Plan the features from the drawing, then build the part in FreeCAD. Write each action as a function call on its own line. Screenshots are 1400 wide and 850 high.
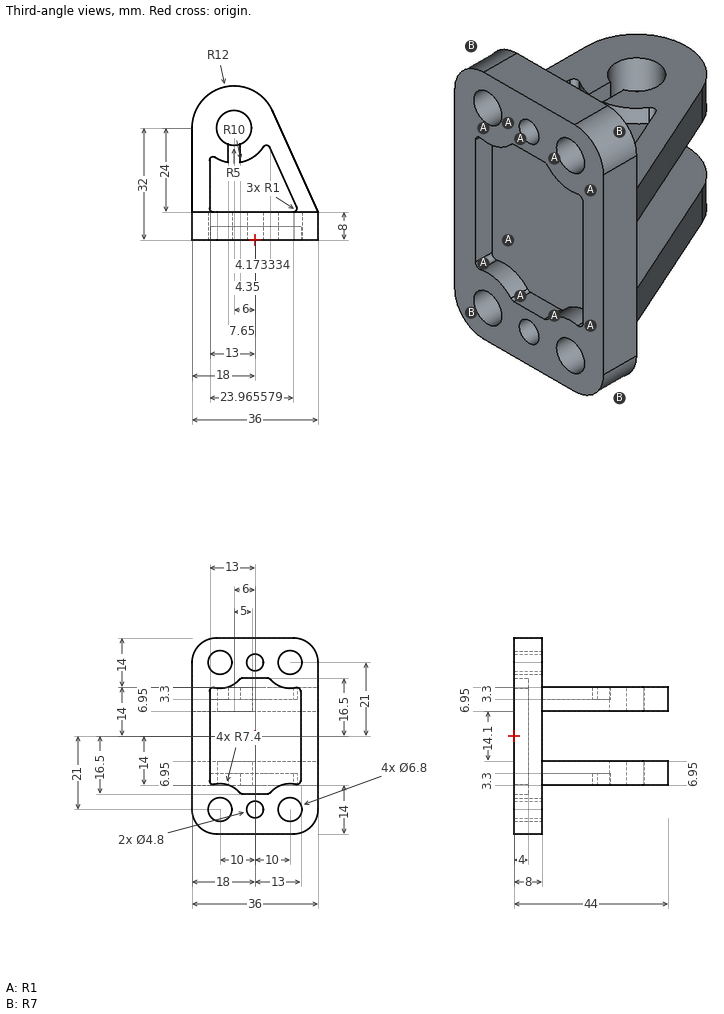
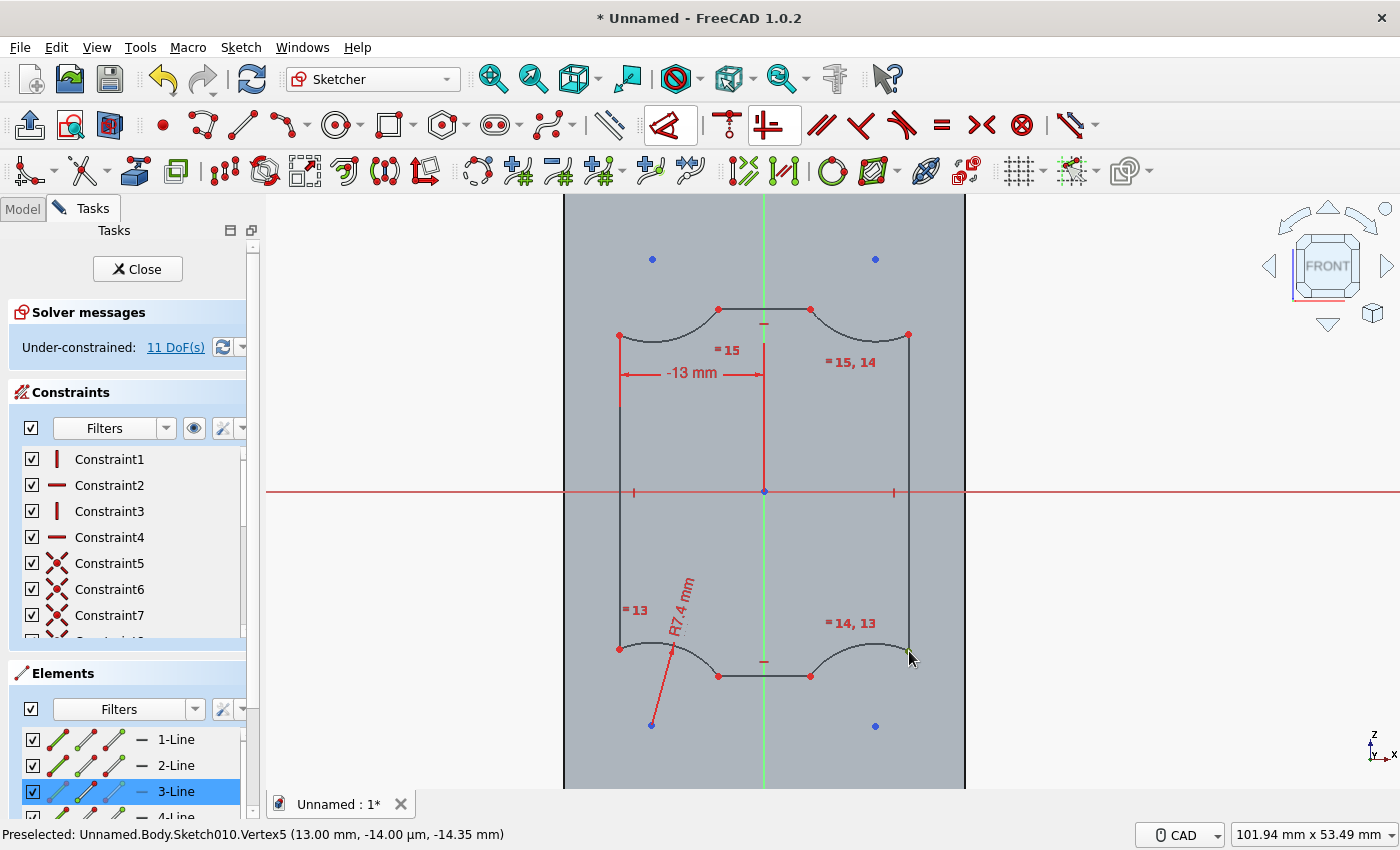
key(l)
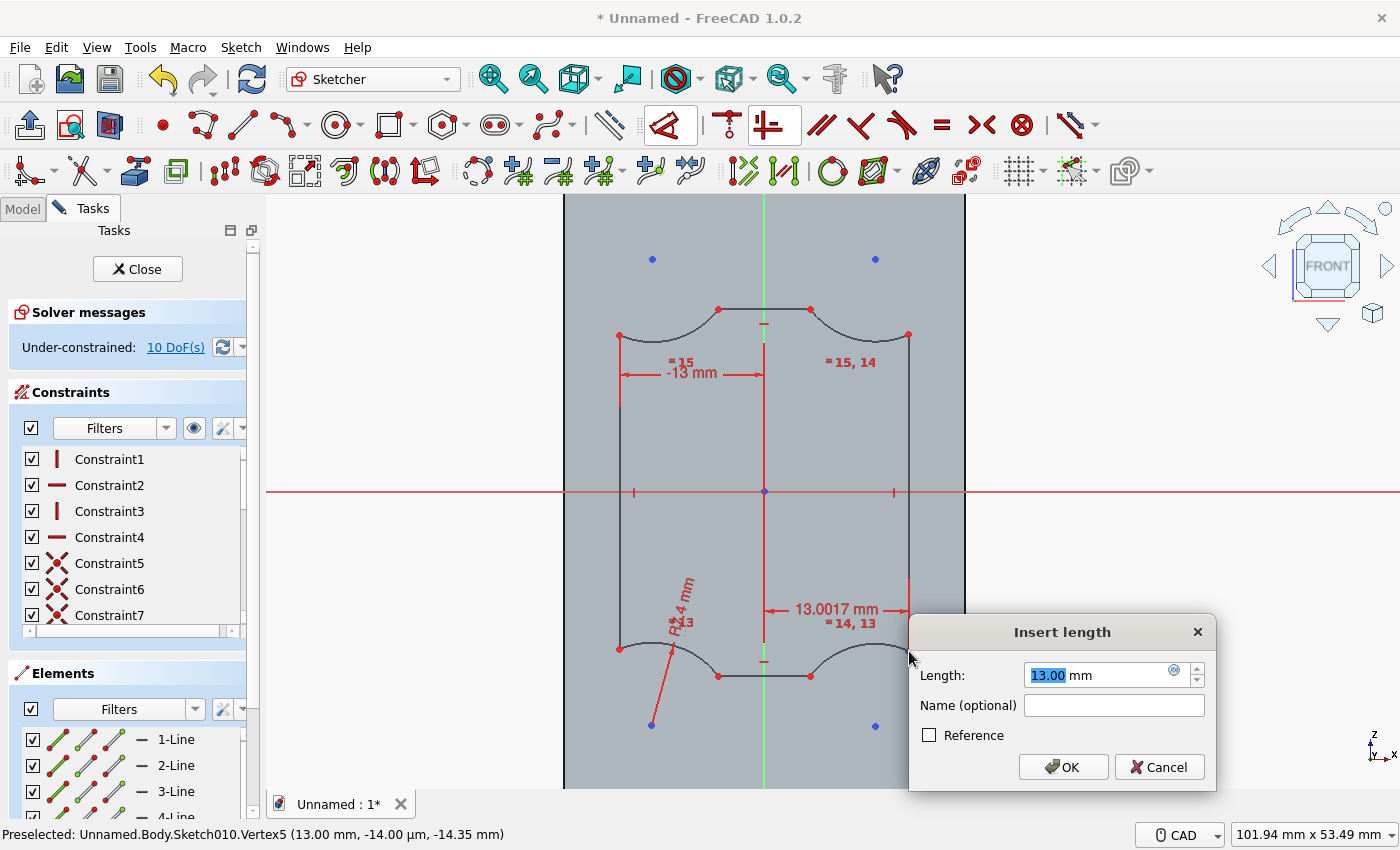
text(13)
key(Return)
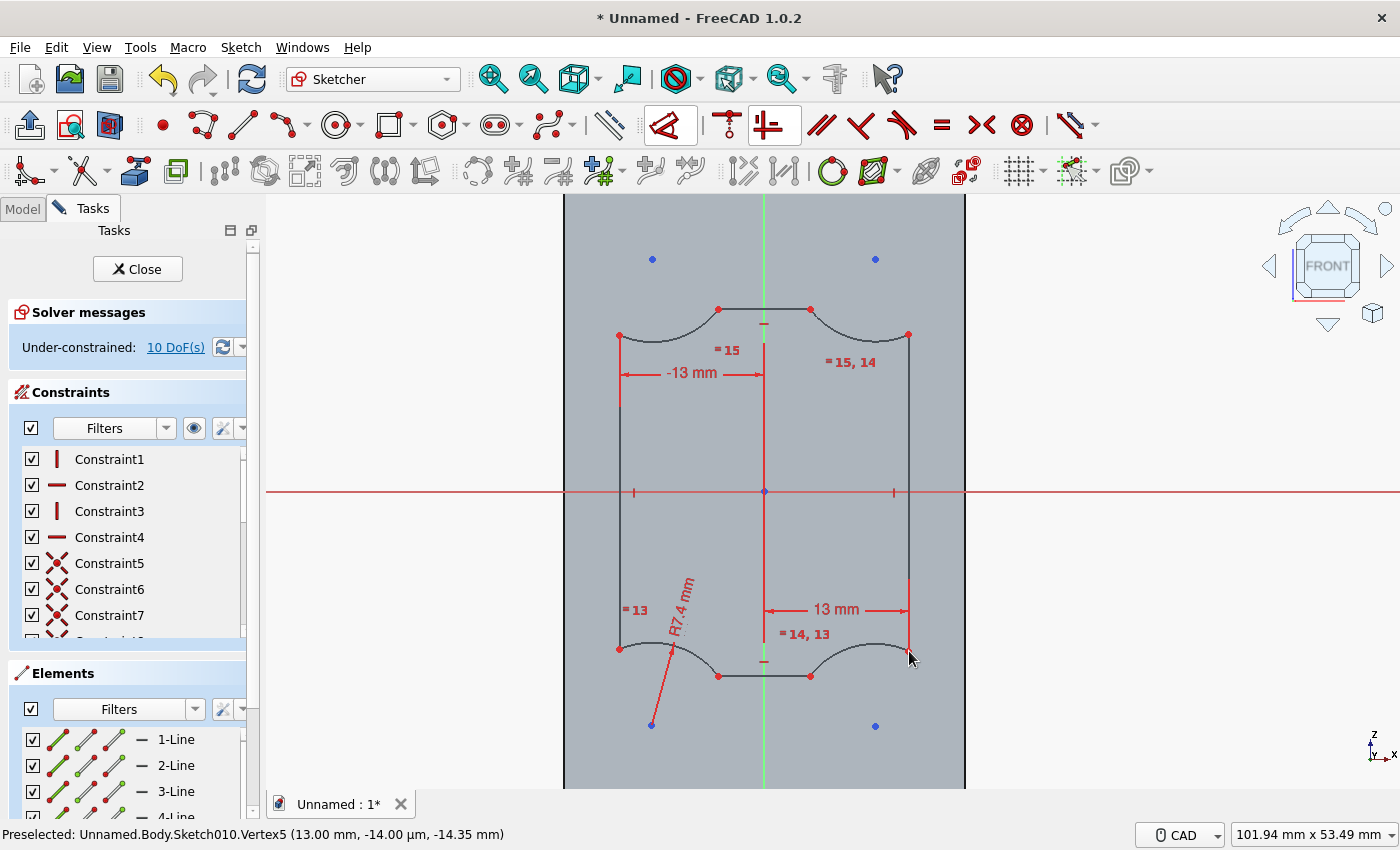
click(652, 725)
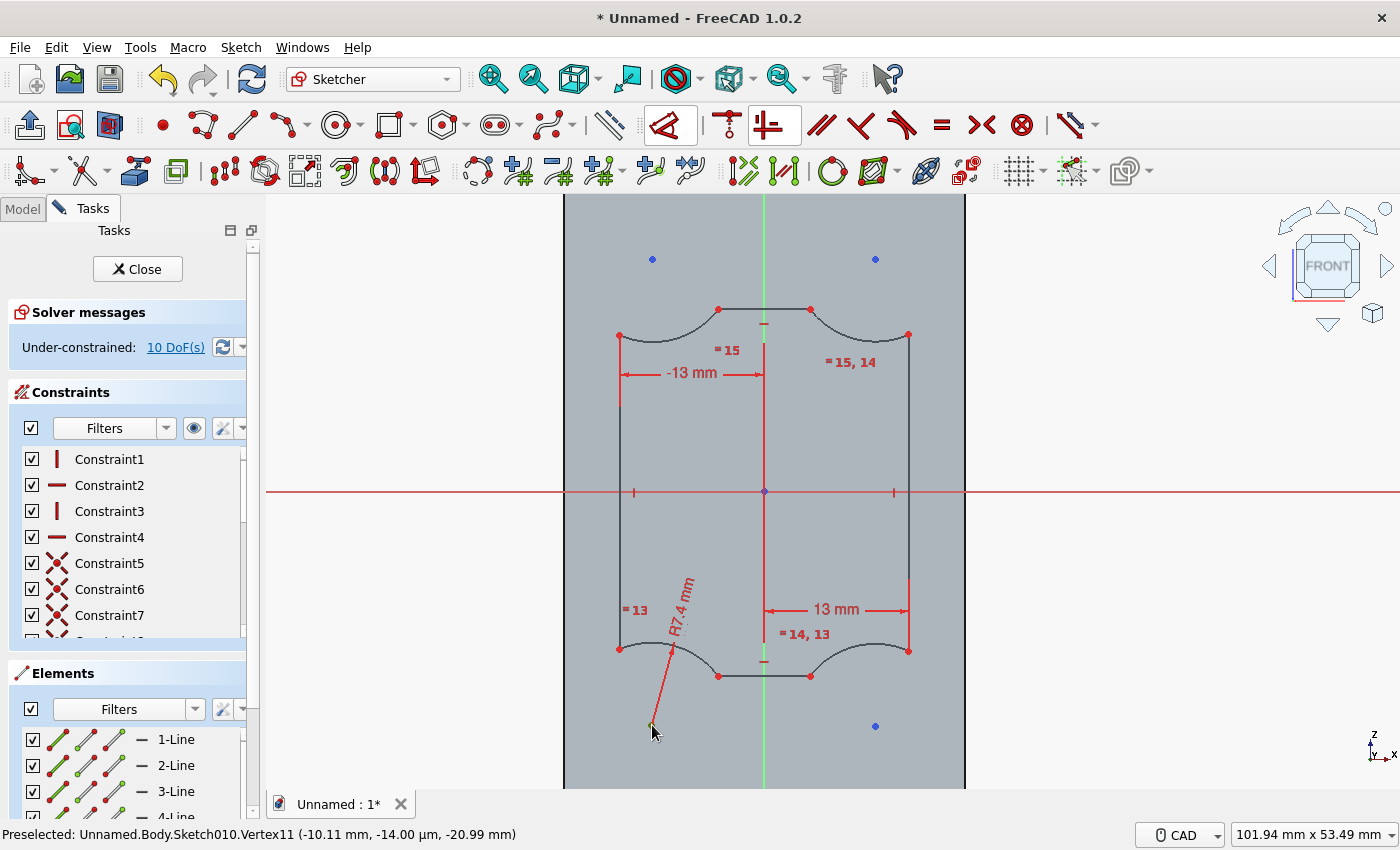
click(692, 126)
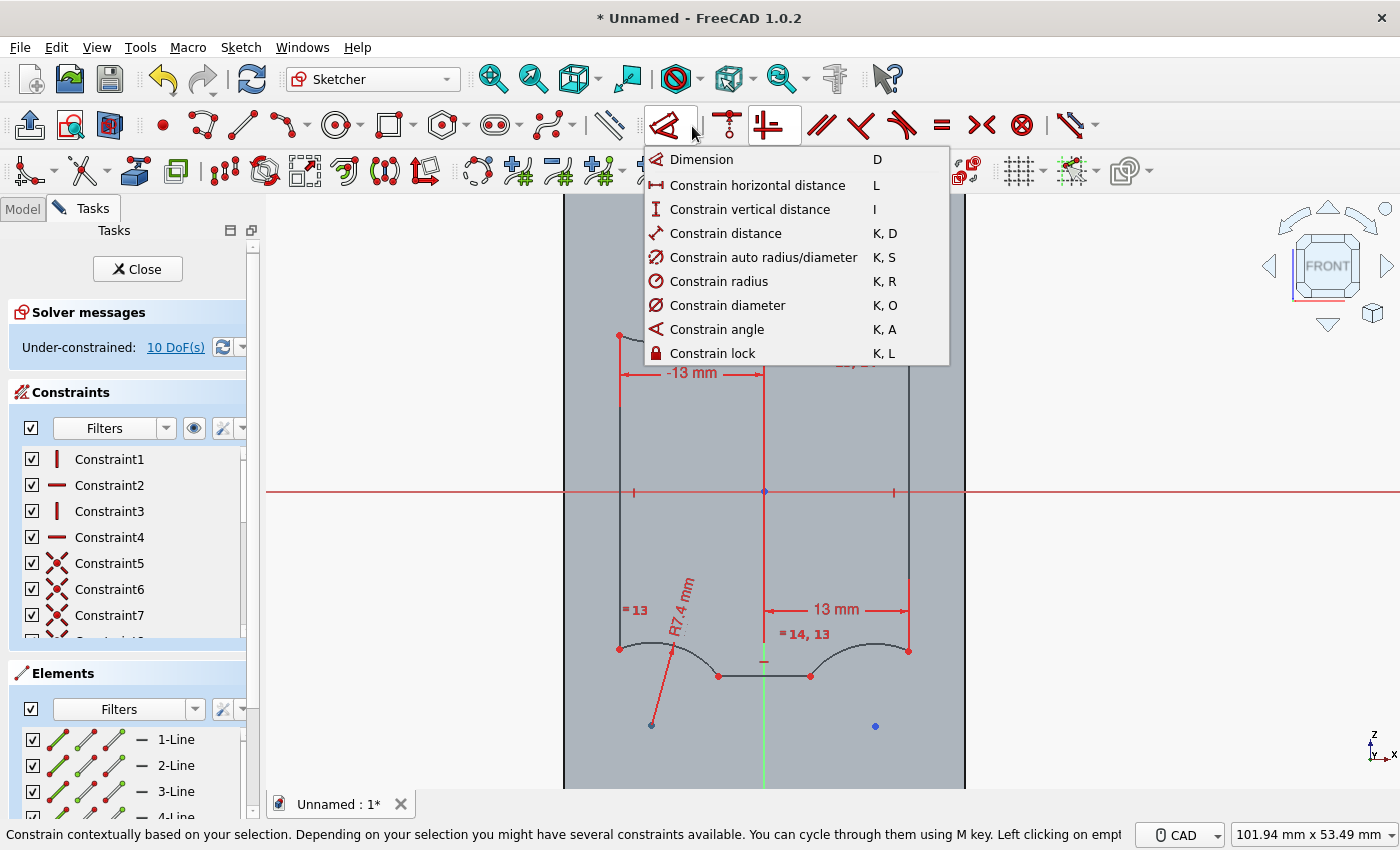
click(797, 185)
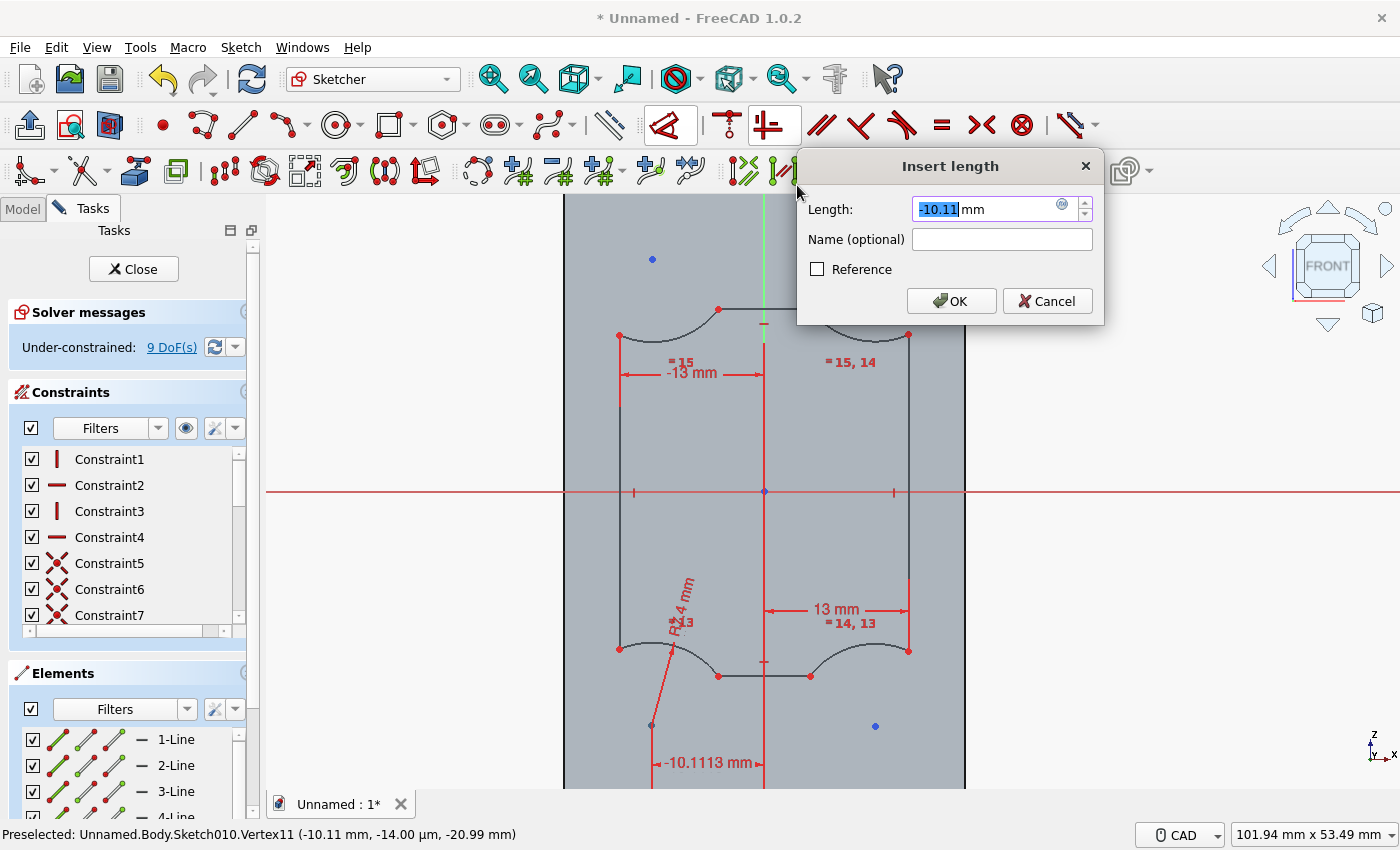
text(-10)
key(Return)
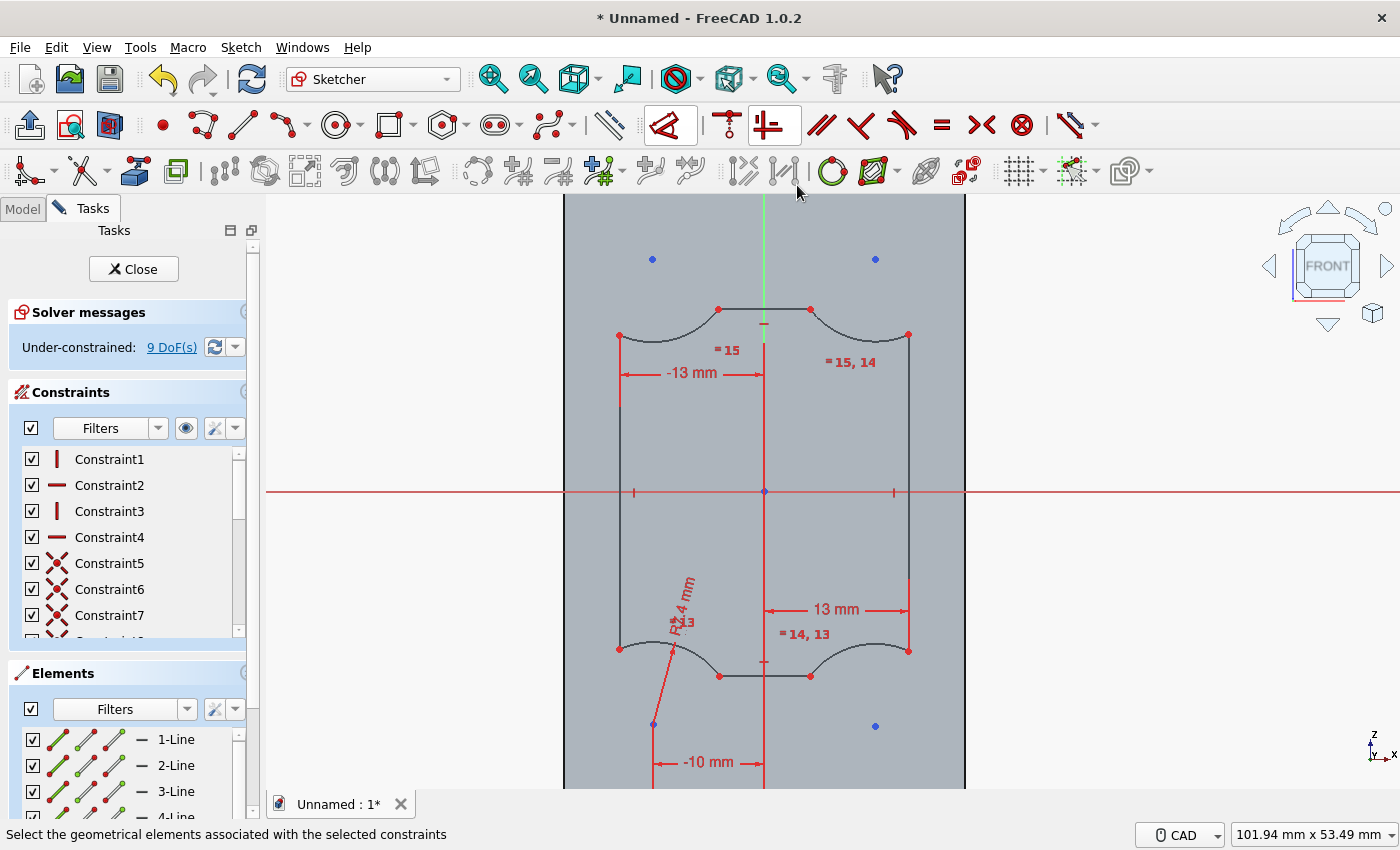
click(653, 725)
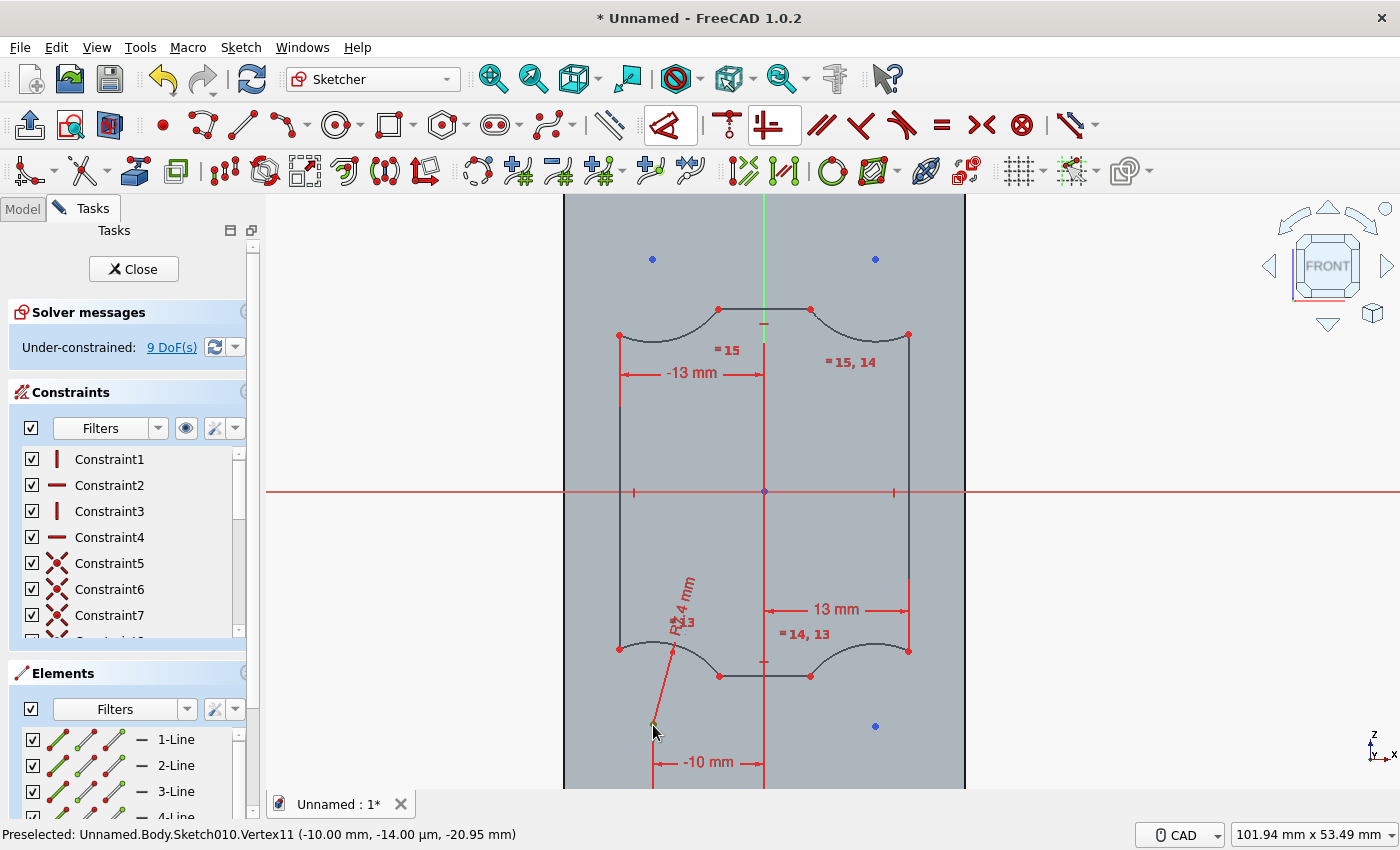
click(692, 126)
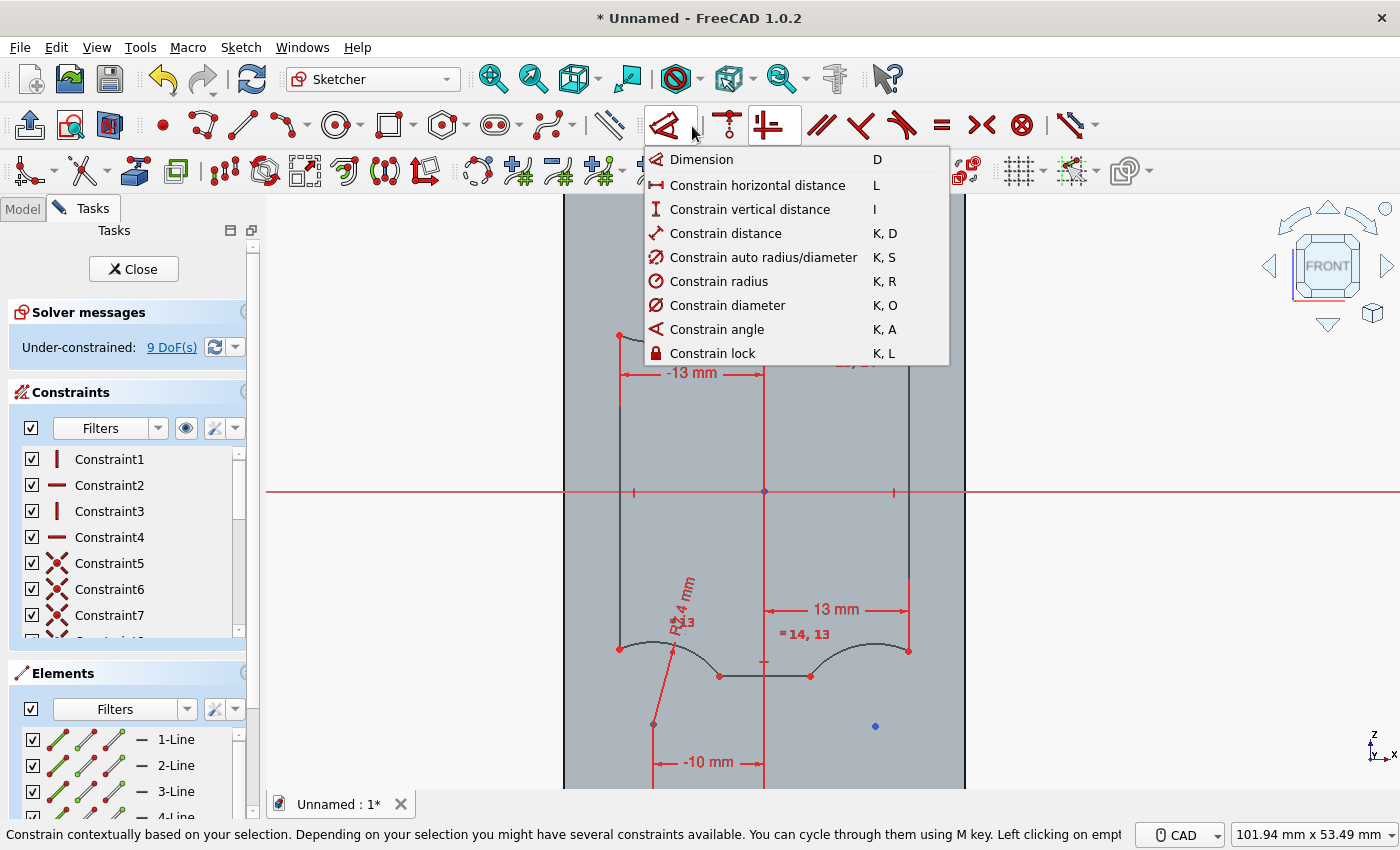
click(797, 209)